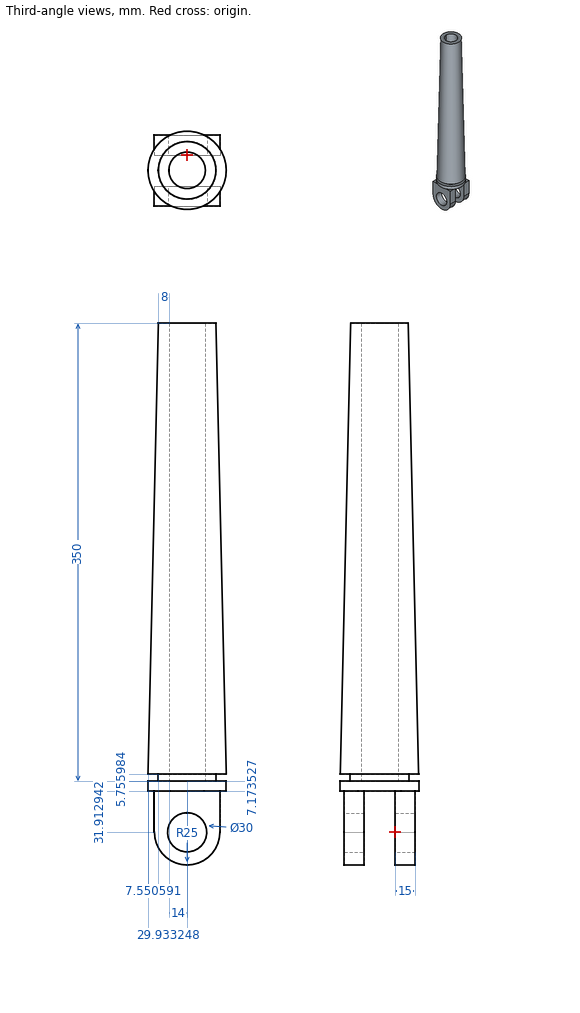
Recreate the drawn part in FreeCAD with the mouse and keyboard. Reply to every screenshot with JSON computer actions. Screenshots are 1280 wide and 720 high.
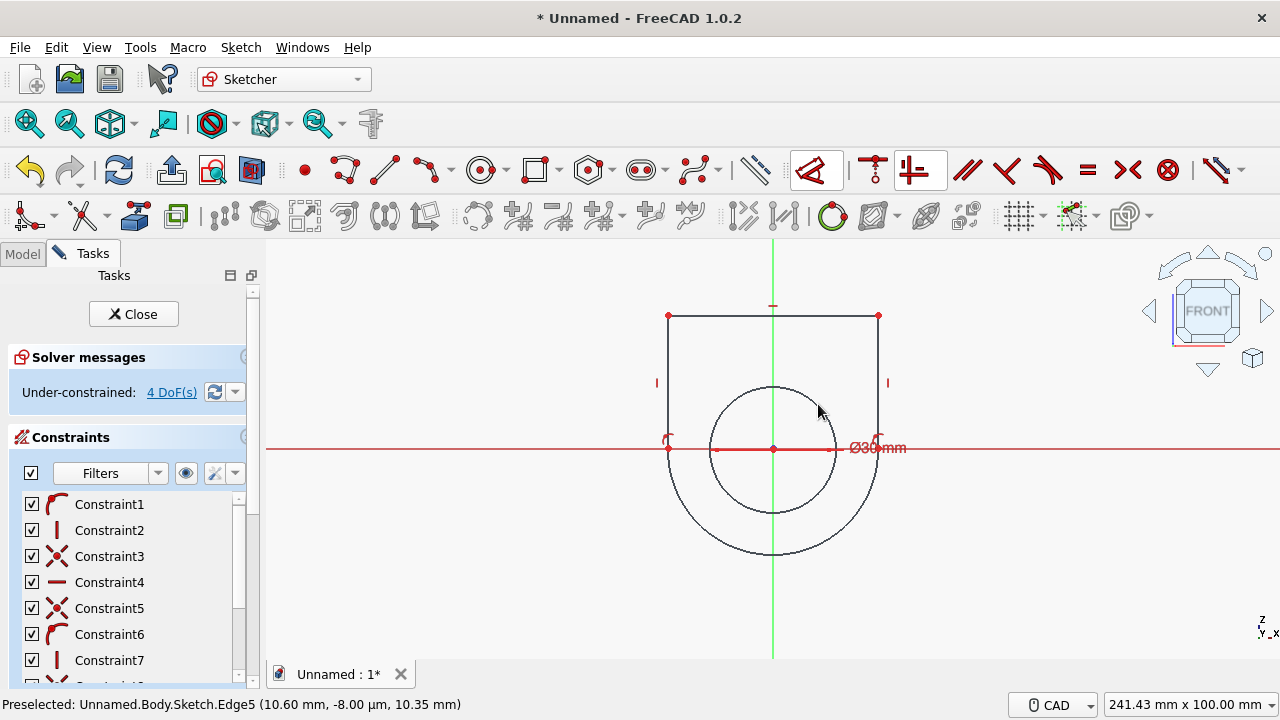
{"action": "left_click", "coordinate": [668, 409]}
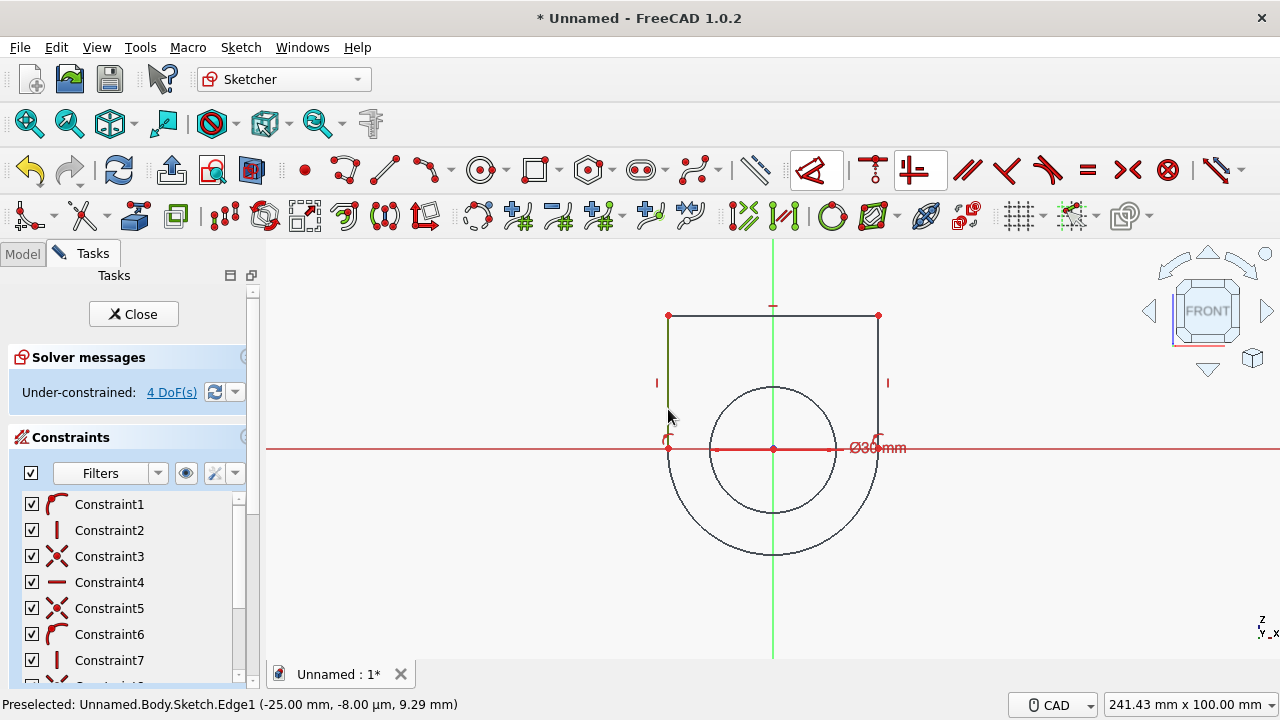
{"action": "left_click", "coordinate": [711, 535]}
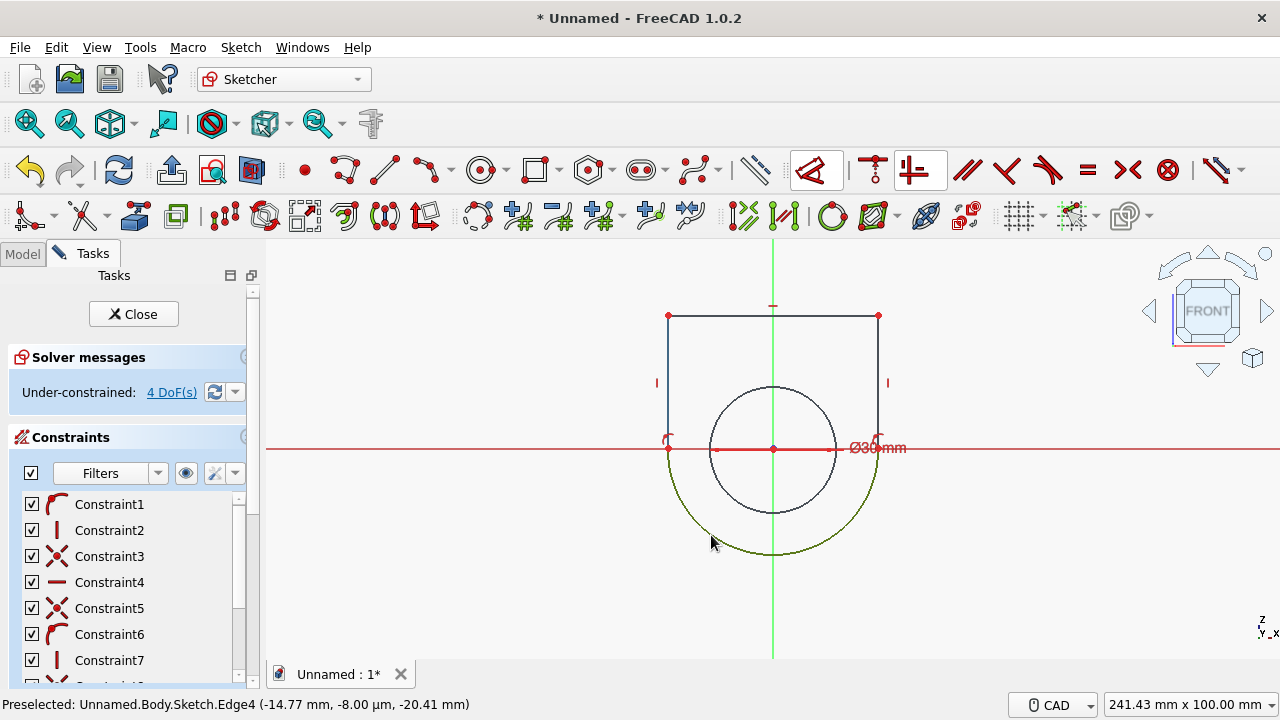
{"action": "left_click", "coordinate": [1048, 170]}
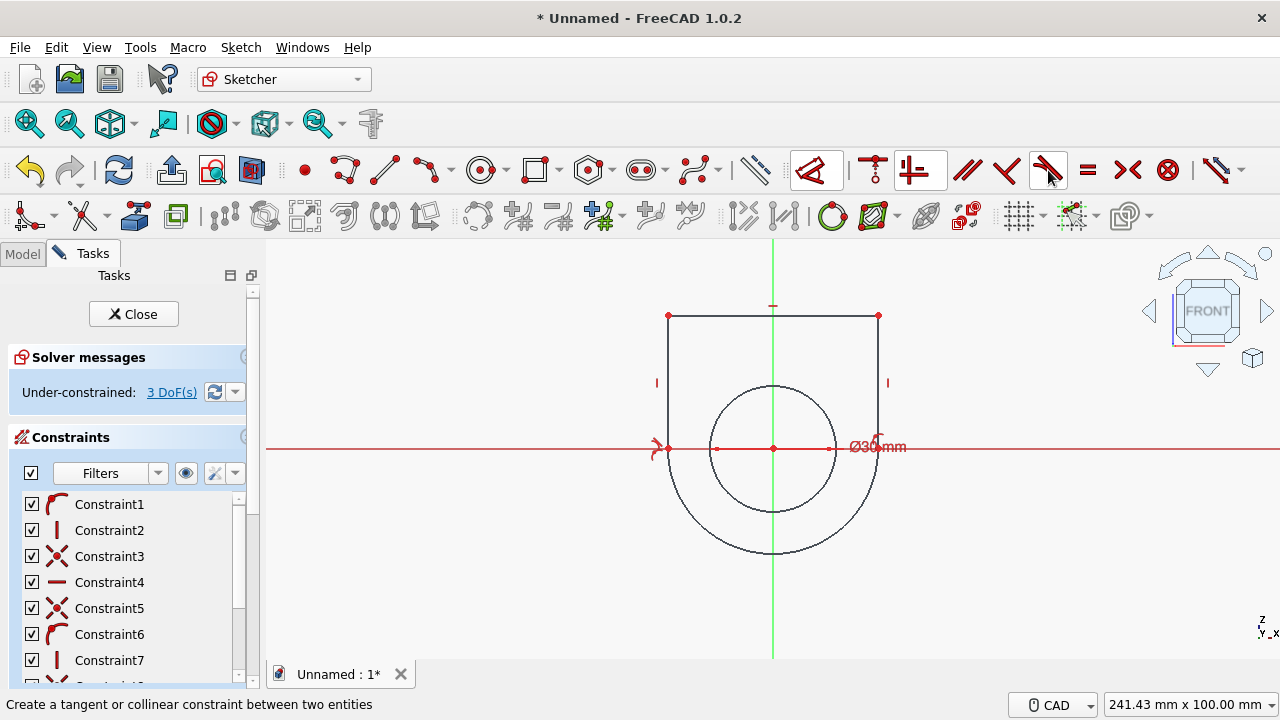
{"action": "left_click", "coordinate": [773, 449]}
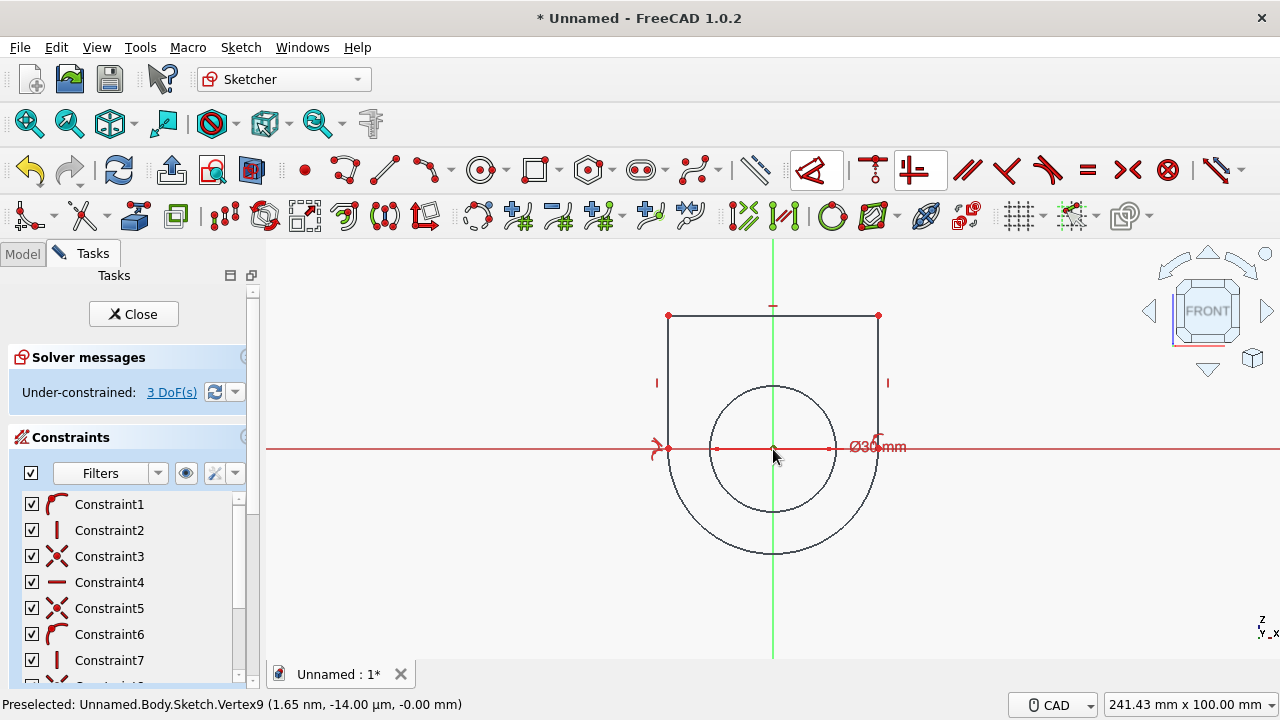
{"action": "left_click", "coordinate": [773, 605]}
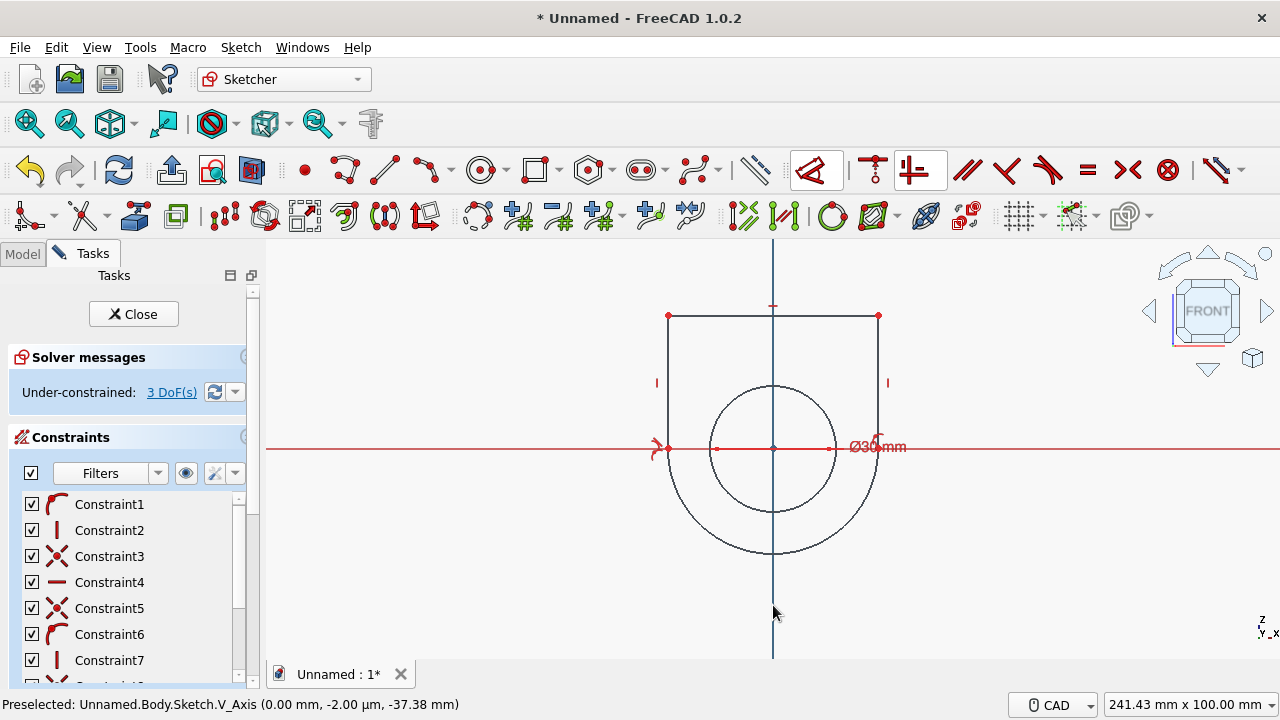
{"action": "left_click", "coordinate": [874, 170]}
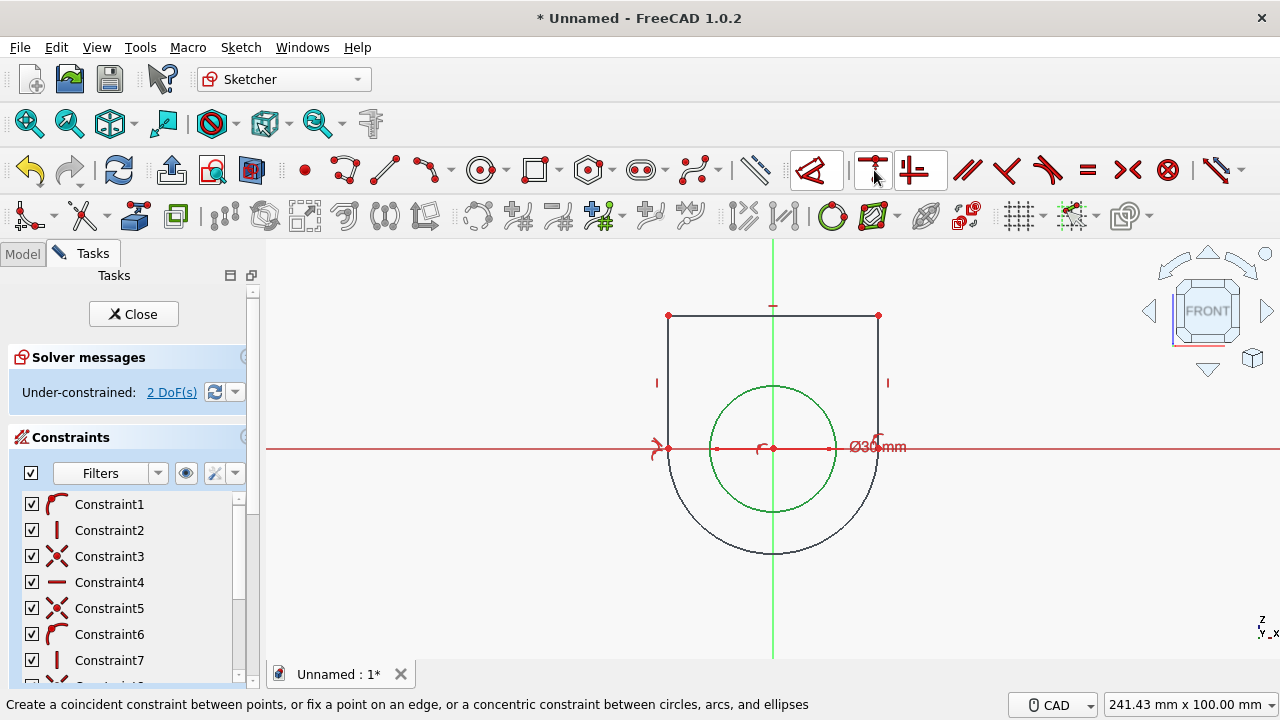
{"action": "left_click", "coordinate": [810, 170]}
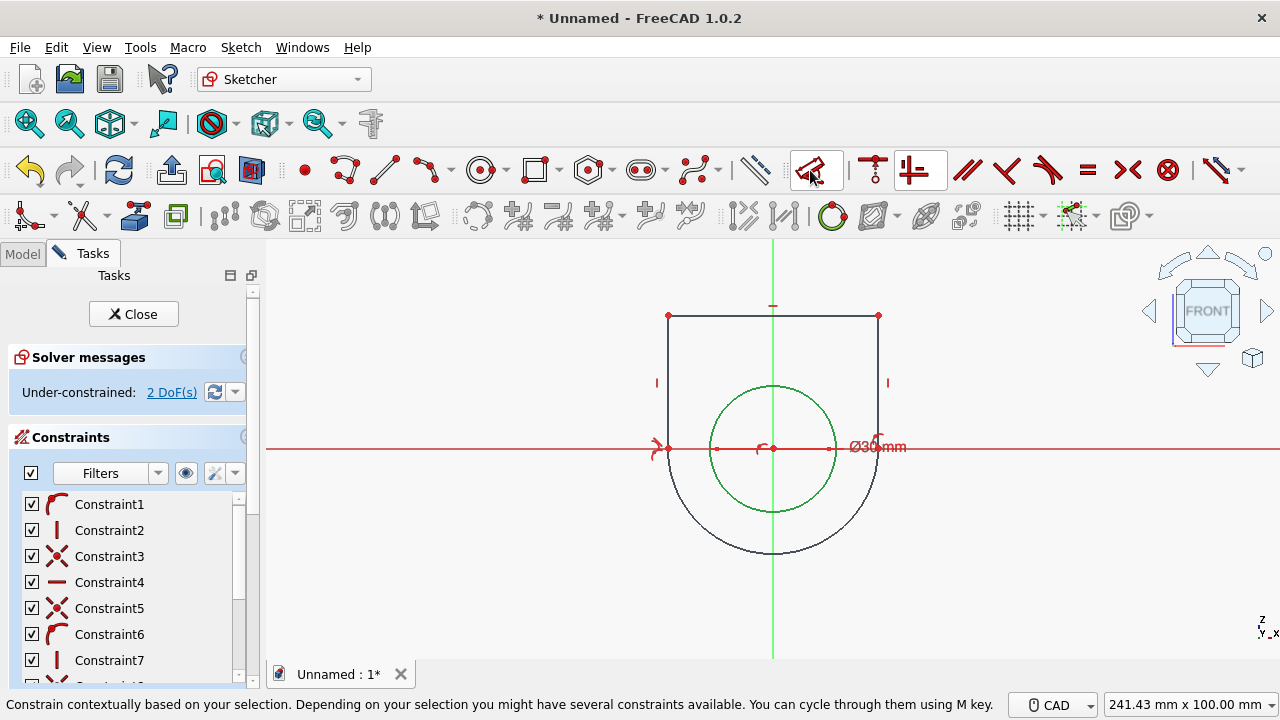
{"action": "left_click", "coordinate": [711, 534]}
{"action": "left_click", "coordinate": [692, 560]}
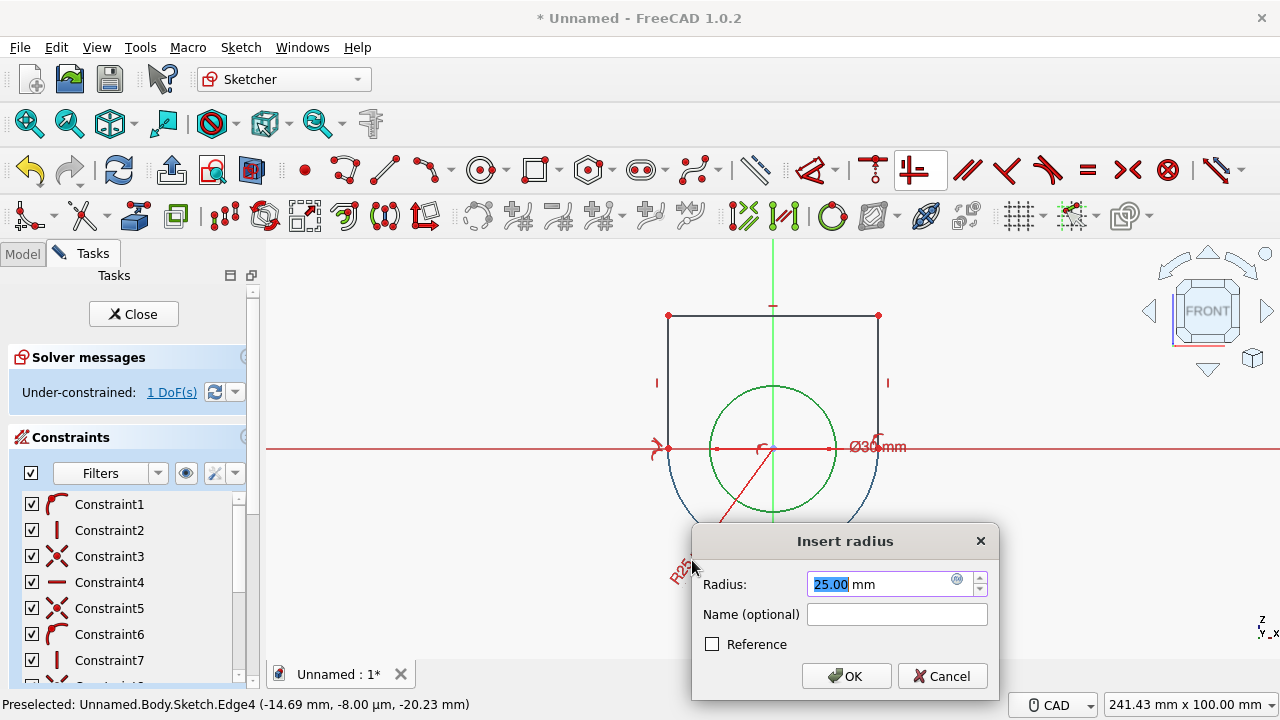
{"action": "type", "text": "25"}
{"action": "key", "text": "Return"}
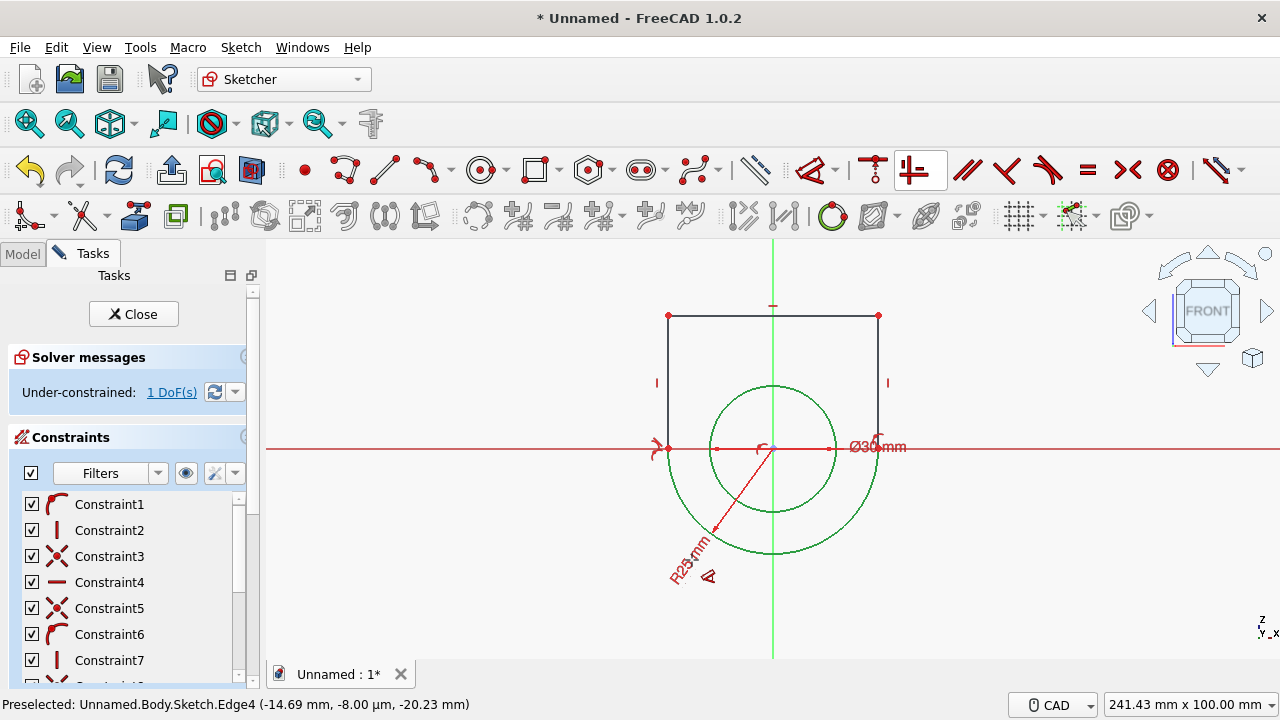
{"action": "left_click", "coordinate": [668, 409]}
{"action": "left_click", "coordinate": [634, 383]}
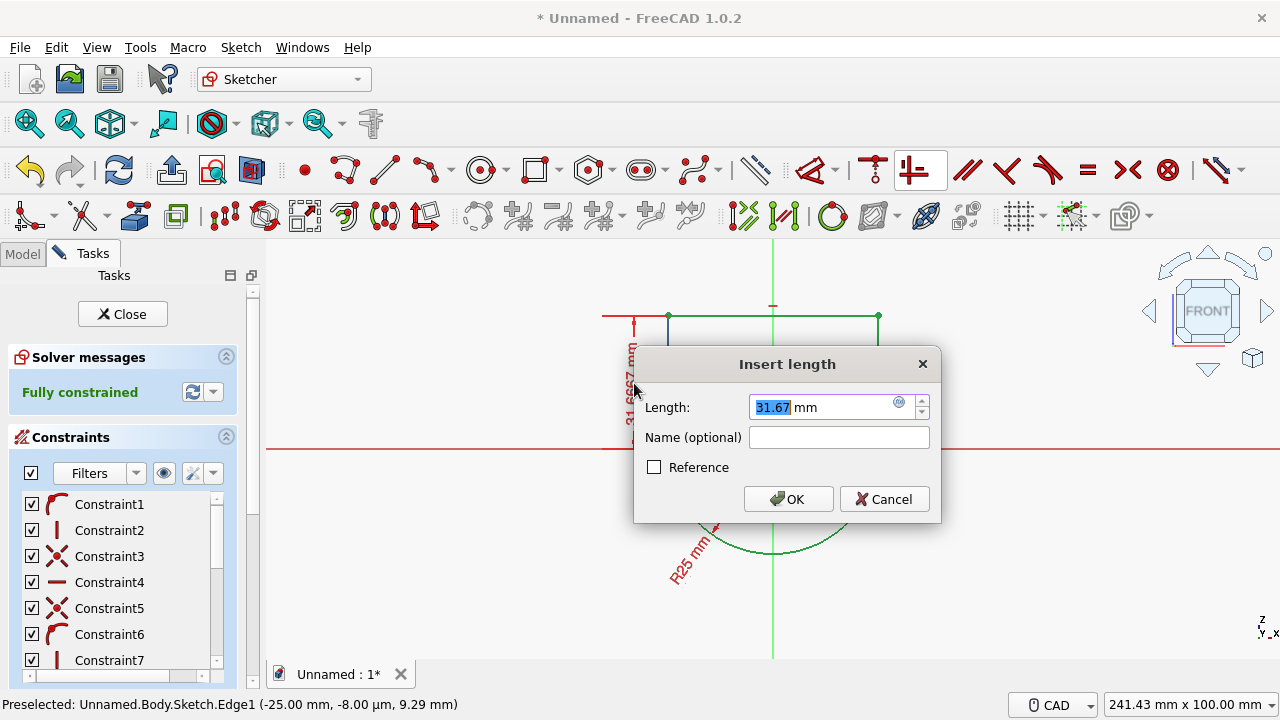
{"action": "type", "text": "31.912942"}
{"action": "key", "text": "Return"}
{"action": "key", "text": "Escape"}